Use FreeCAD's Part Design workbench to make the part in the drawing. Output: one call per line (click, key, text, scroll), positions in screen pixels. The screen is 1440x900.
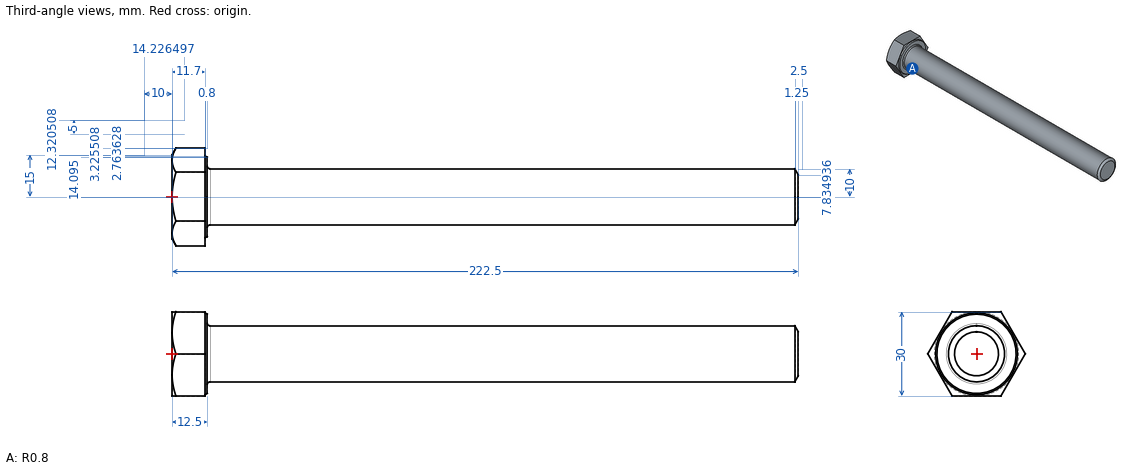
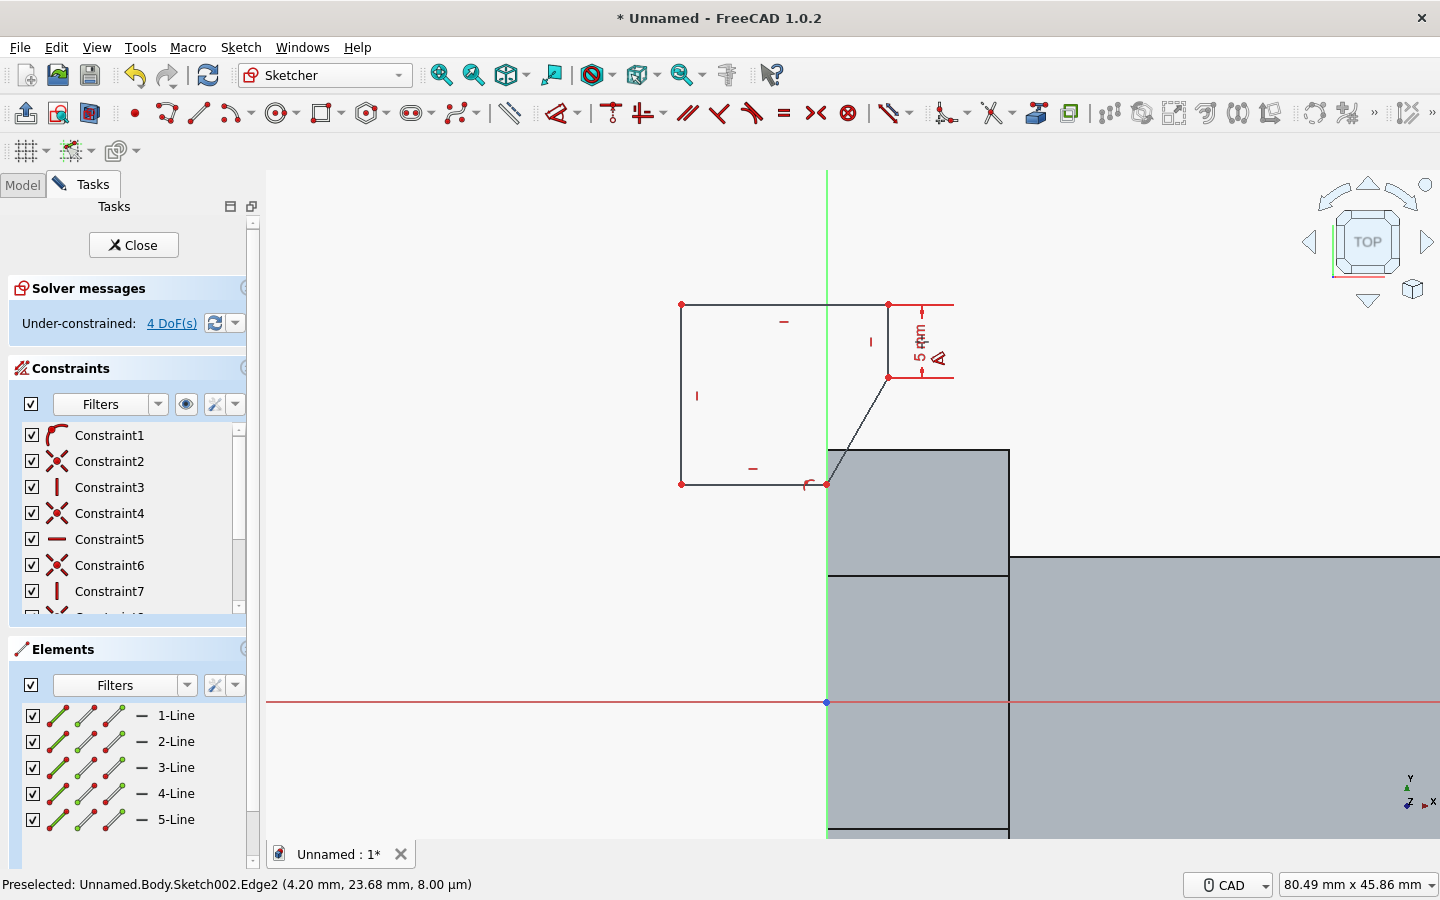
click(725, 485)
click(754, 451)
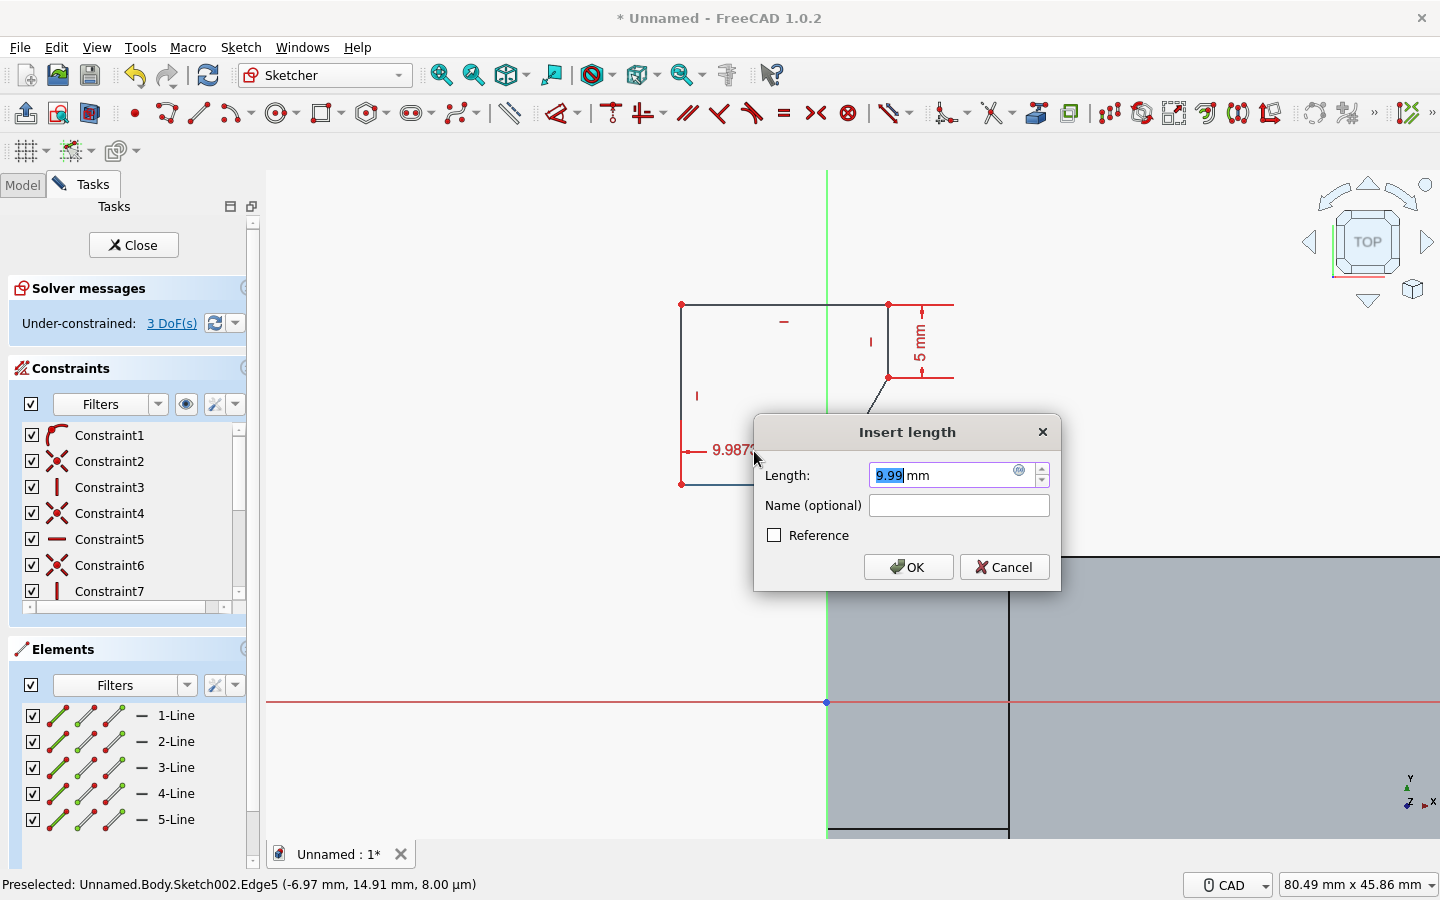
text(10)
key(Return)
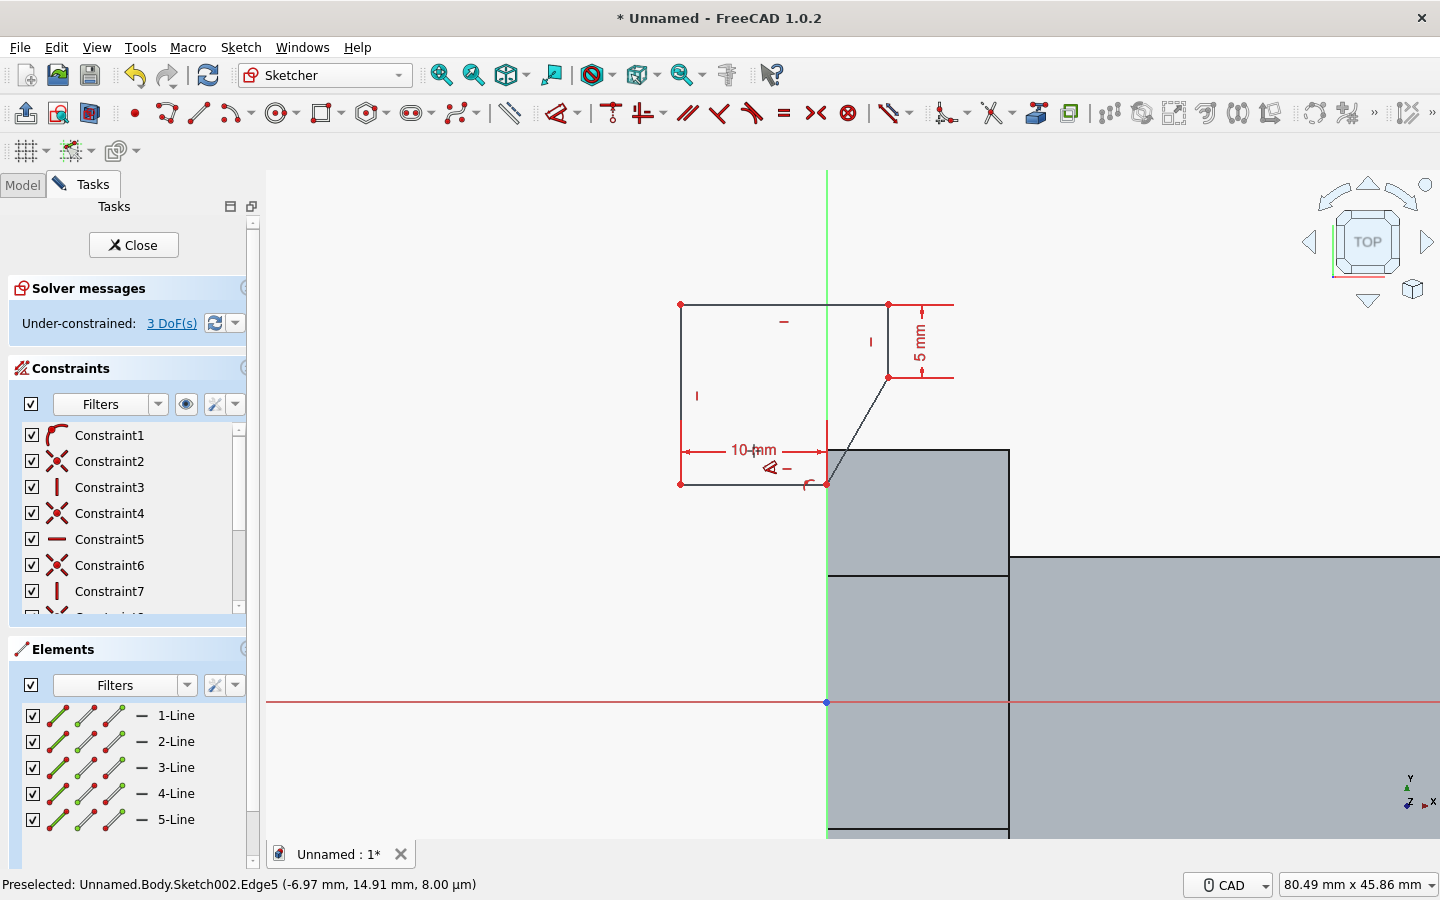
click(827, 485)
click(861, 594)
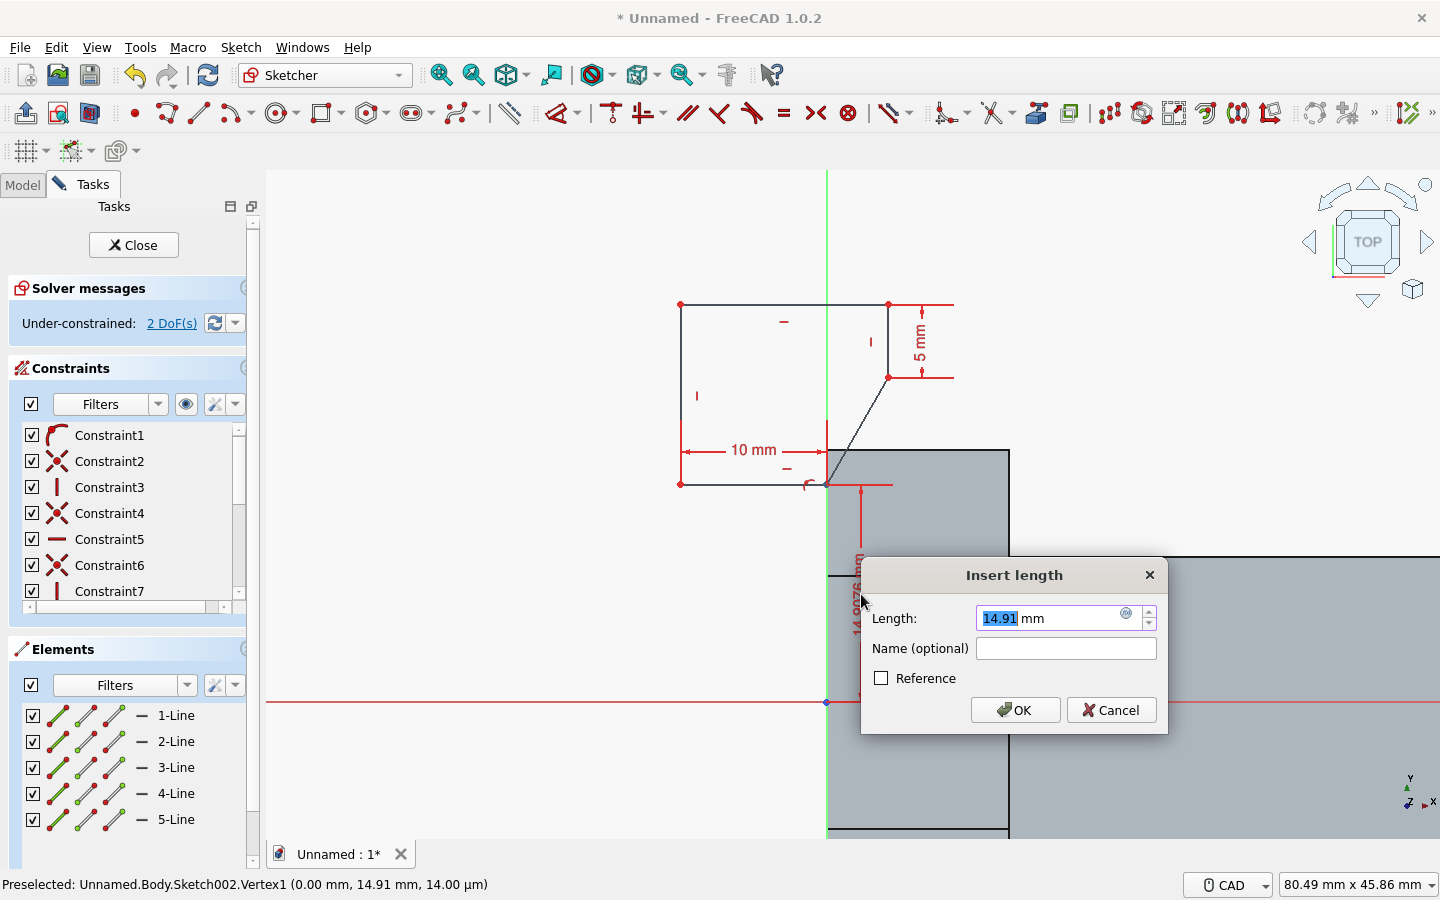
text(15)
key(Return)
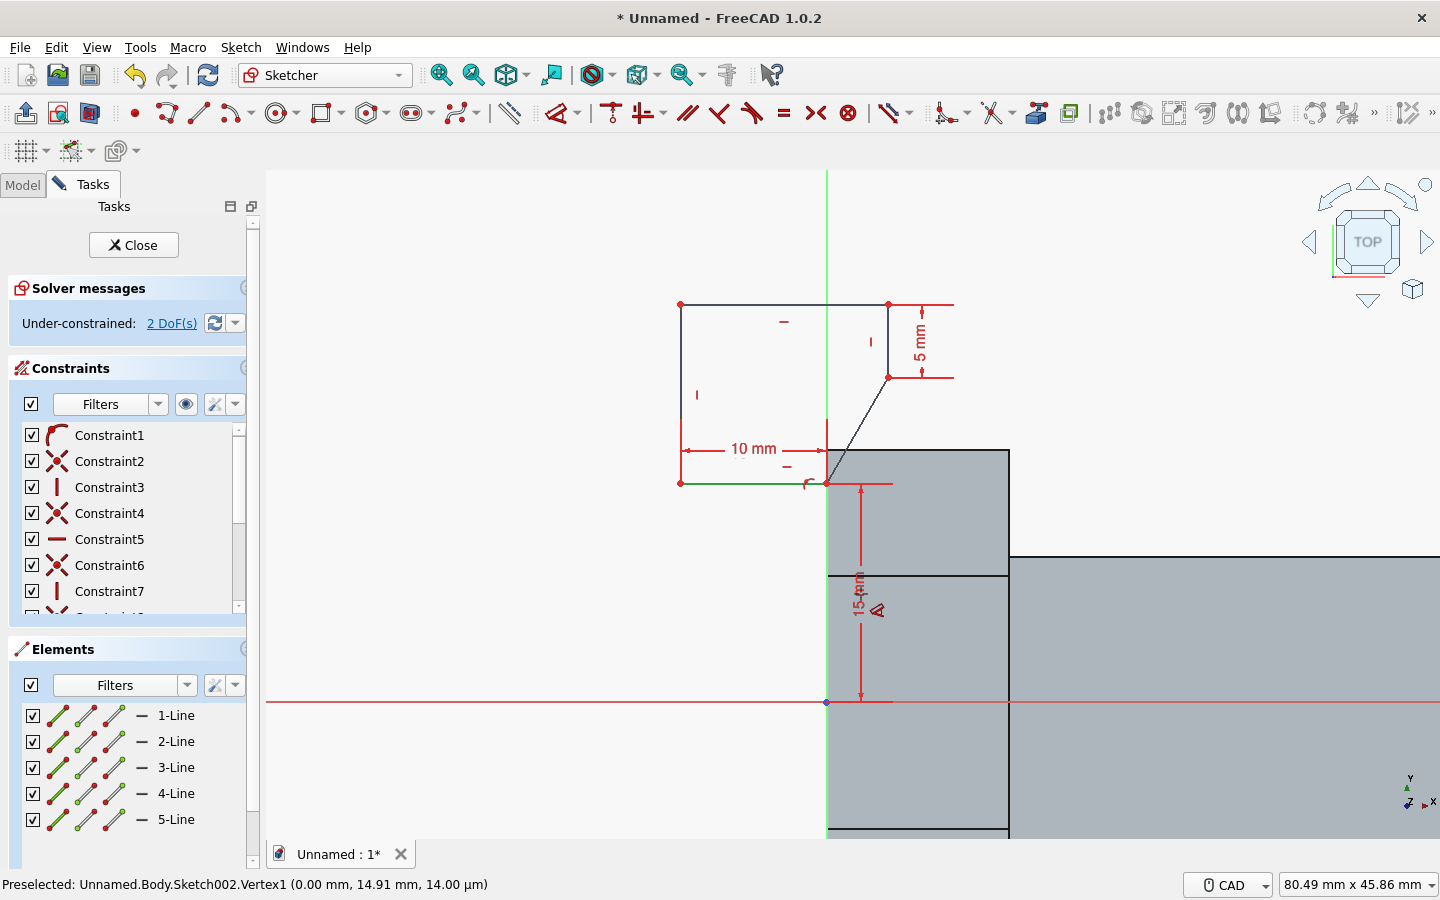
click(826, 305)
click(784, 271)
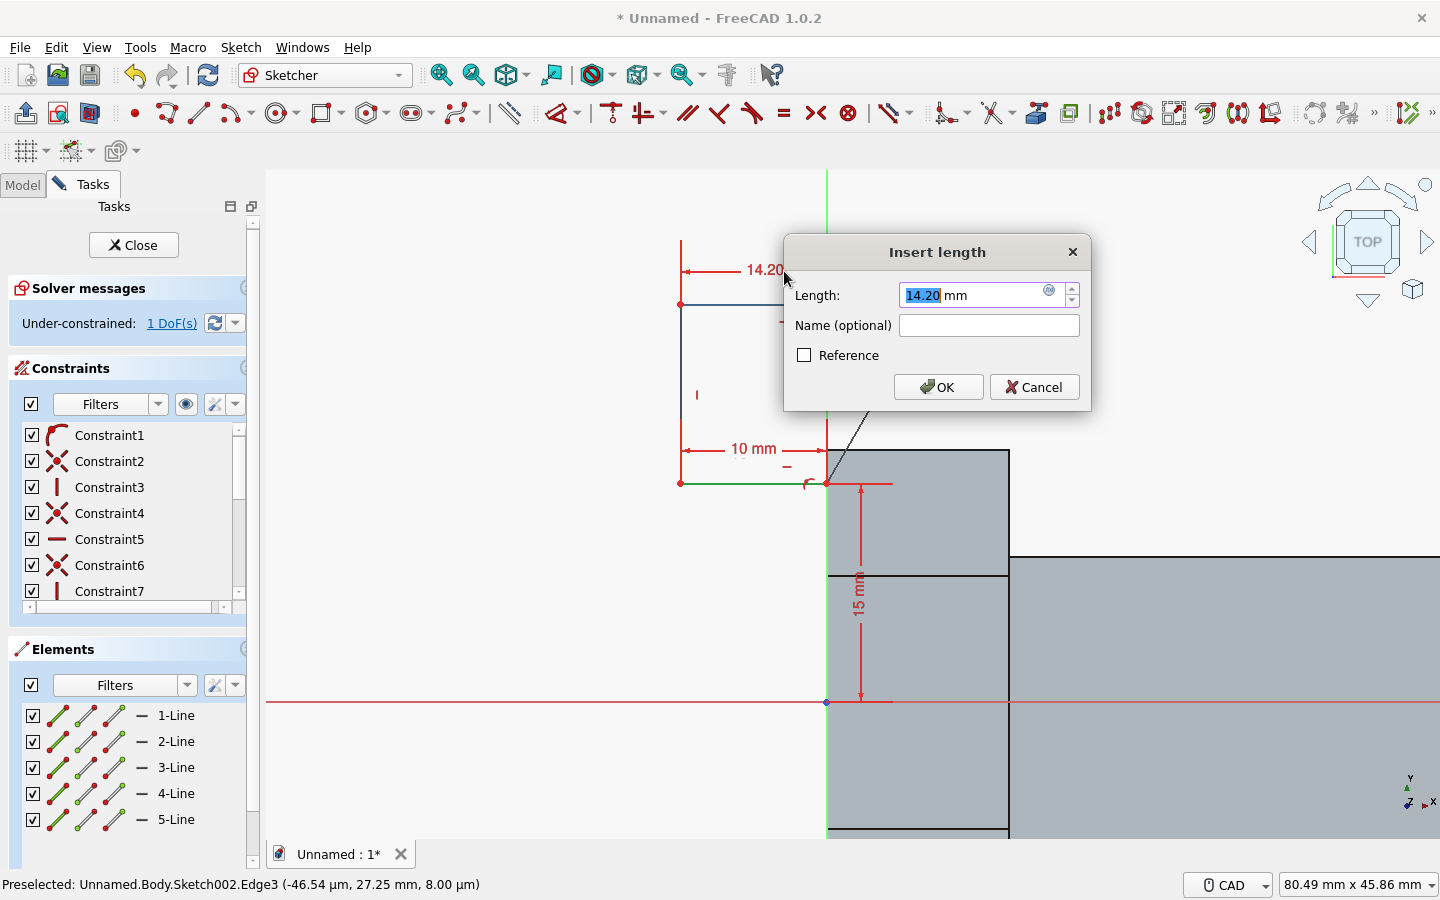
text(14.226497)
key(Return)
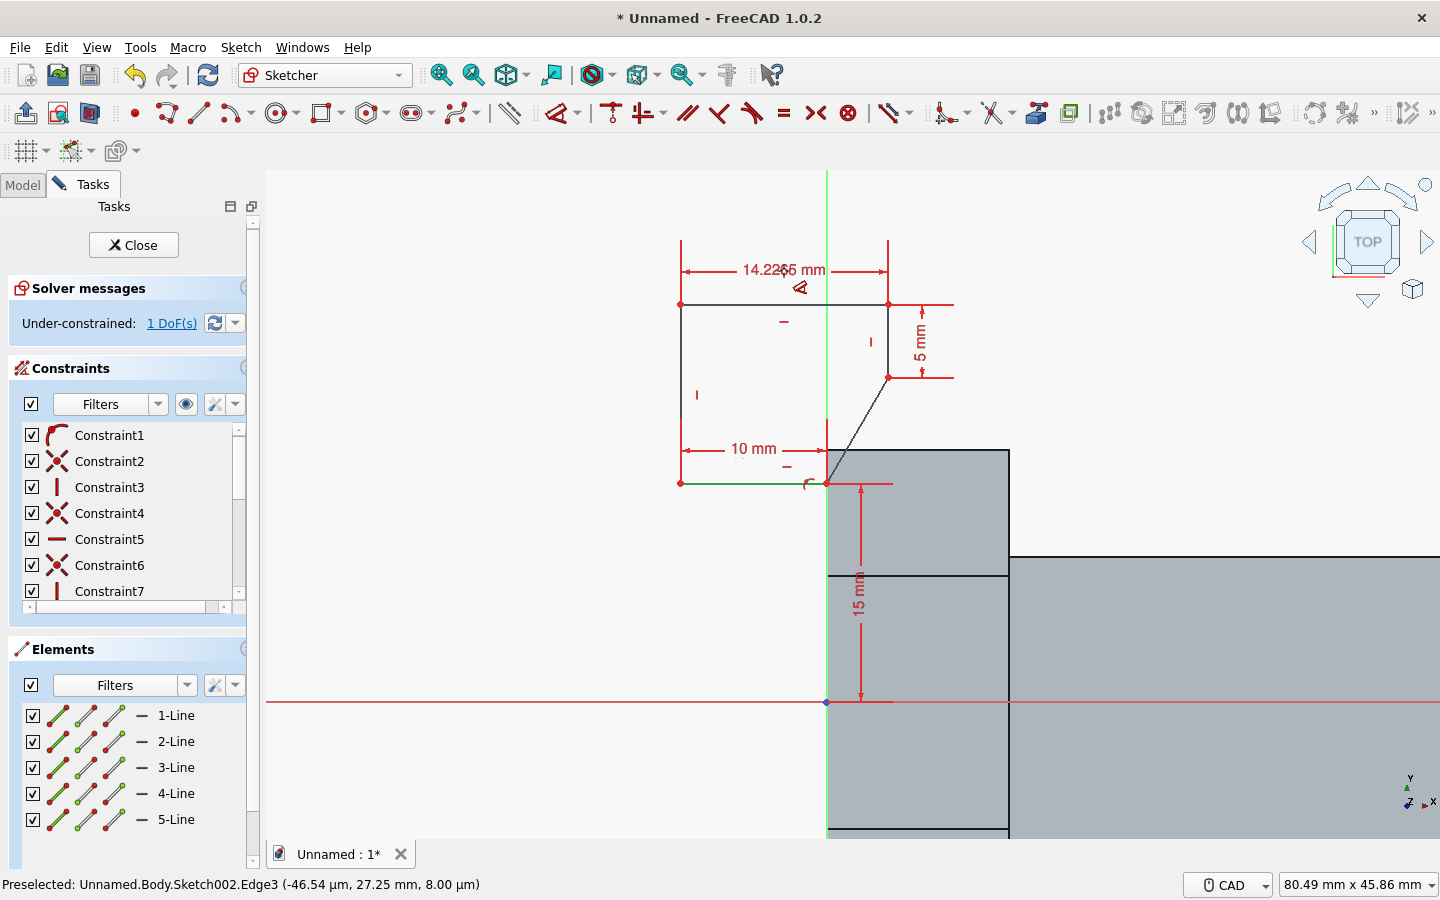
click(681, 359)
click(647, 394)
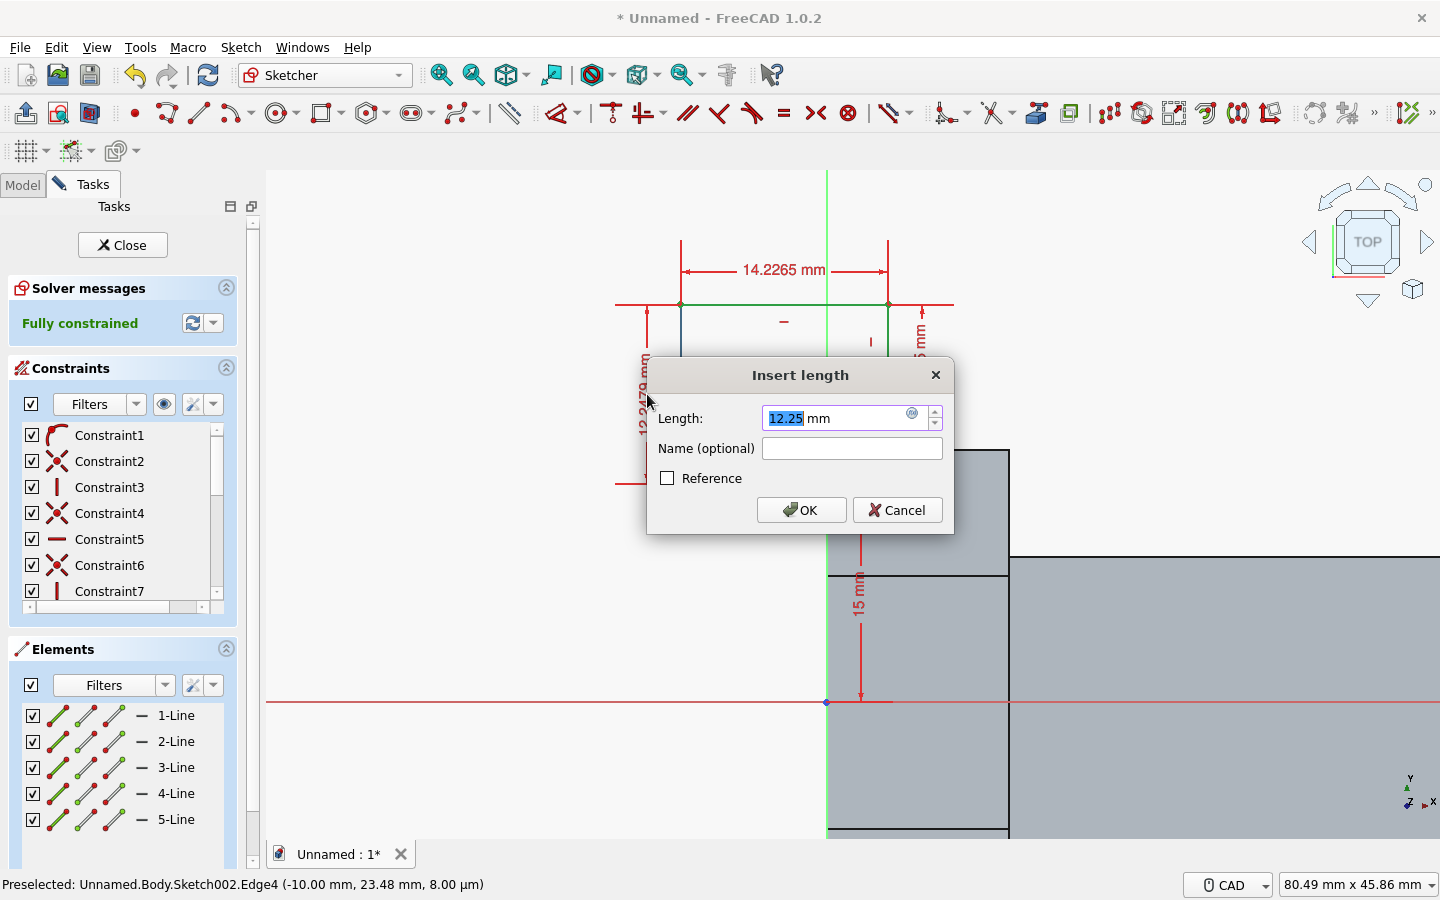
text(12.320508)
key(Return)
key(Escape)